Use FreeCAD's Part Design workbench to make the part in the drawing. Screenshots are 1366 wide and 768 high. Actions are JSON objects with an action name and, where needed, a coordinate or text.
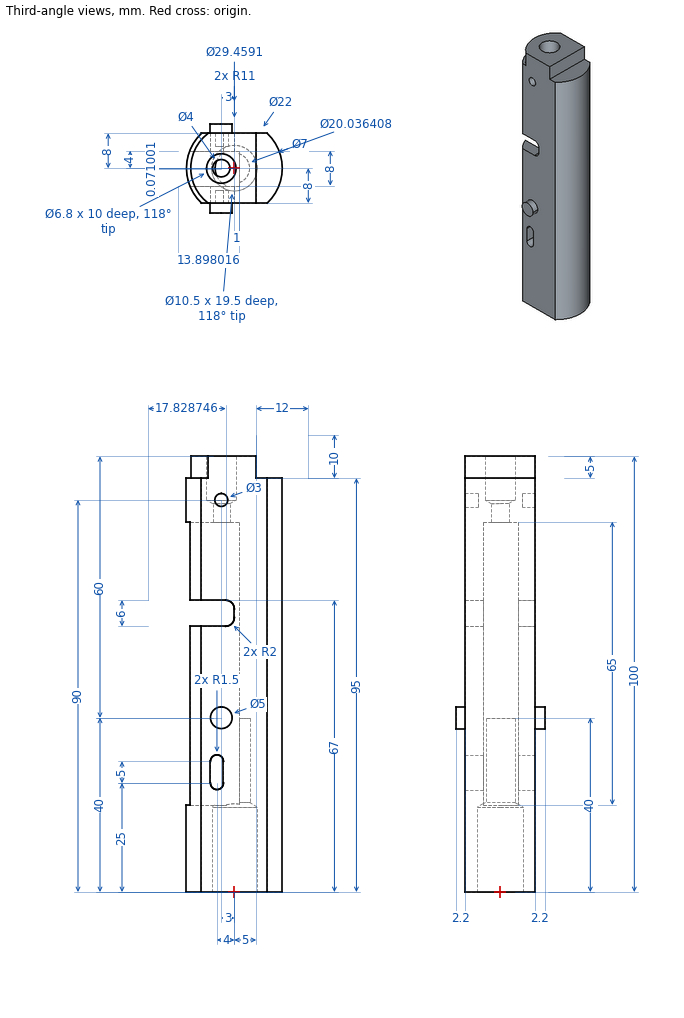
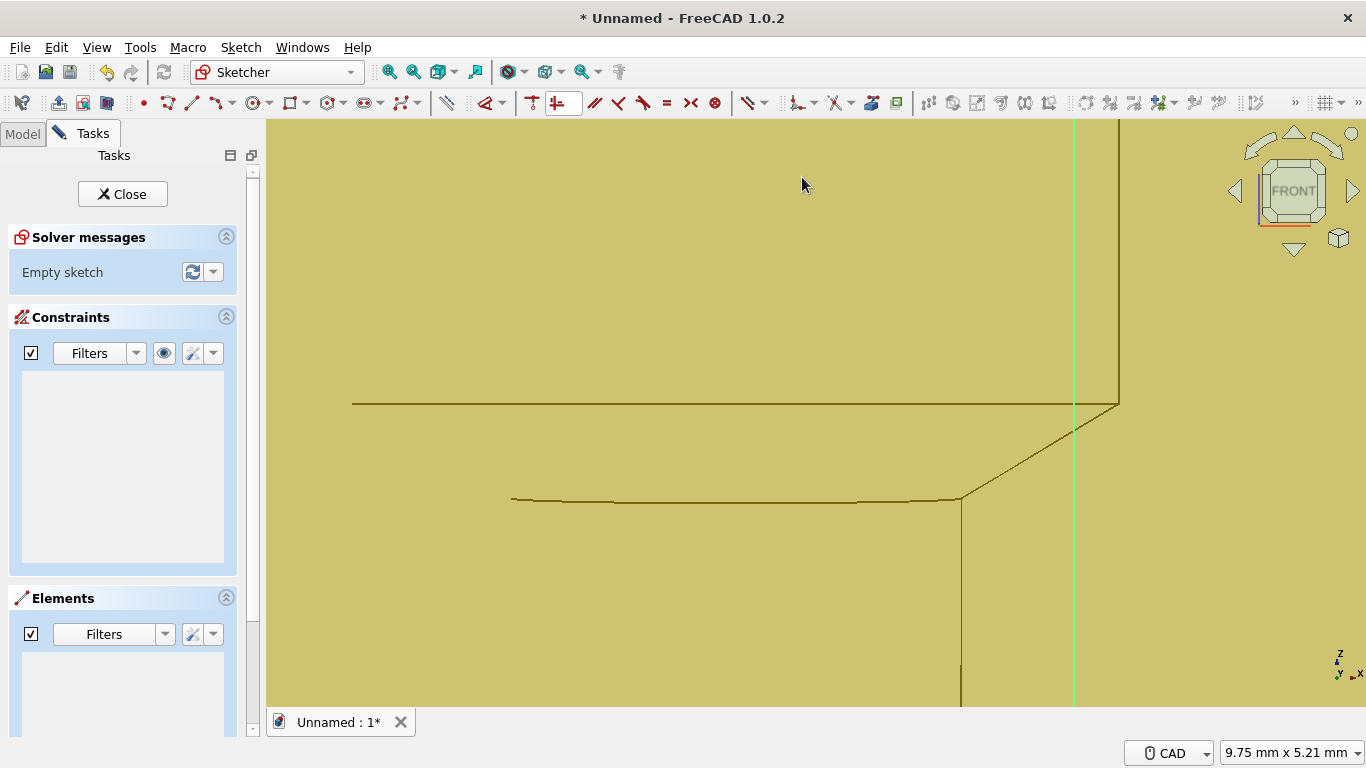
{"action": "key", "text": "g c"}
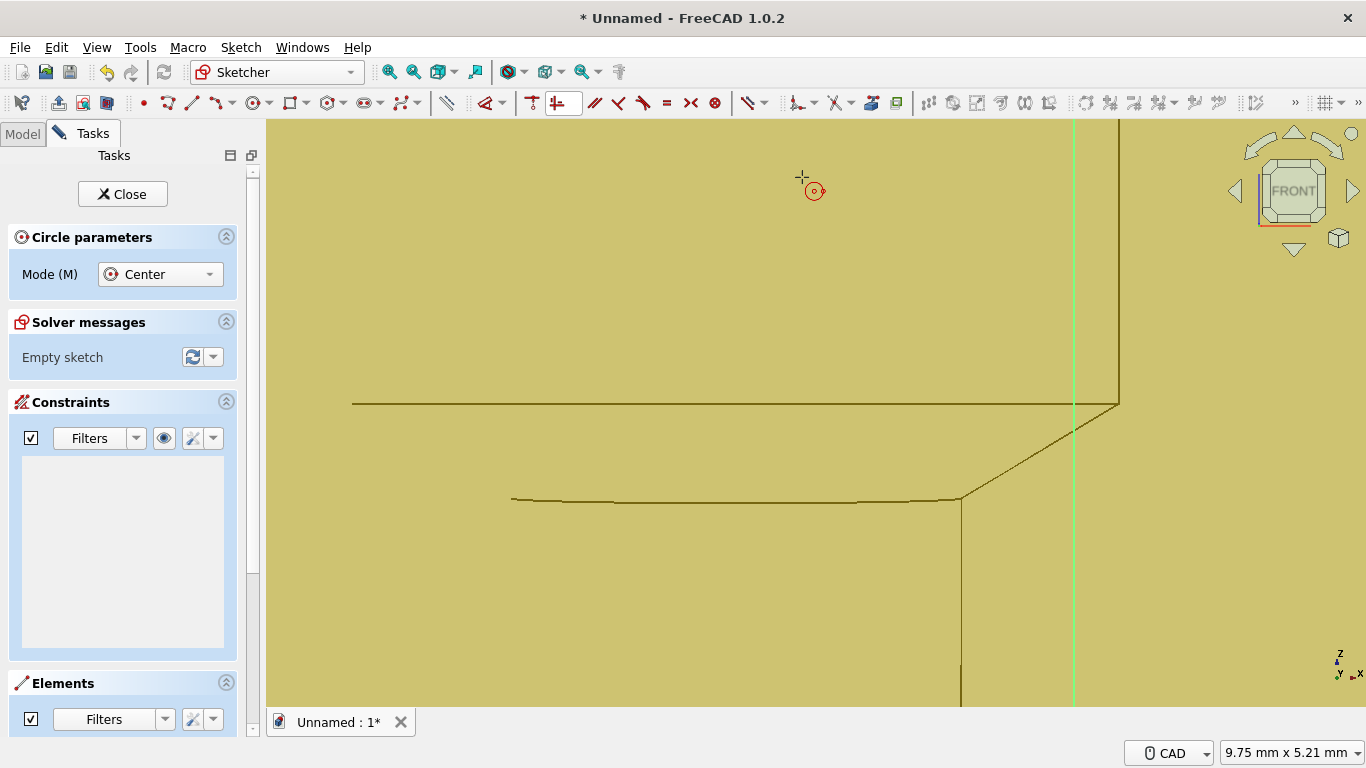
{"action": "left_click", "coordinate": [736, 404]}
{"action": "mouse_move", "coordinate": [855, 284]}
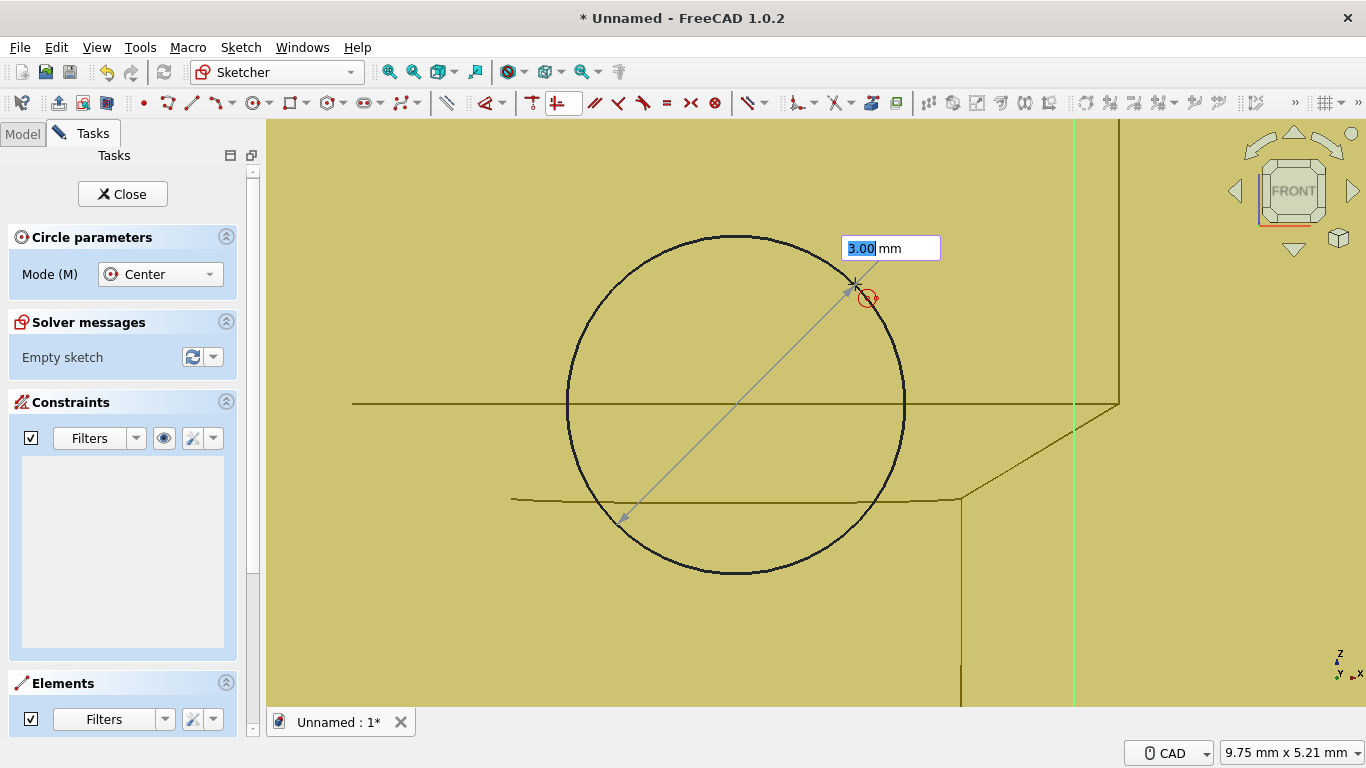
{"action": "type", "text": "3"}
{"action": "key", "text": "Return"}
{"action": "key", "text": "Escape"}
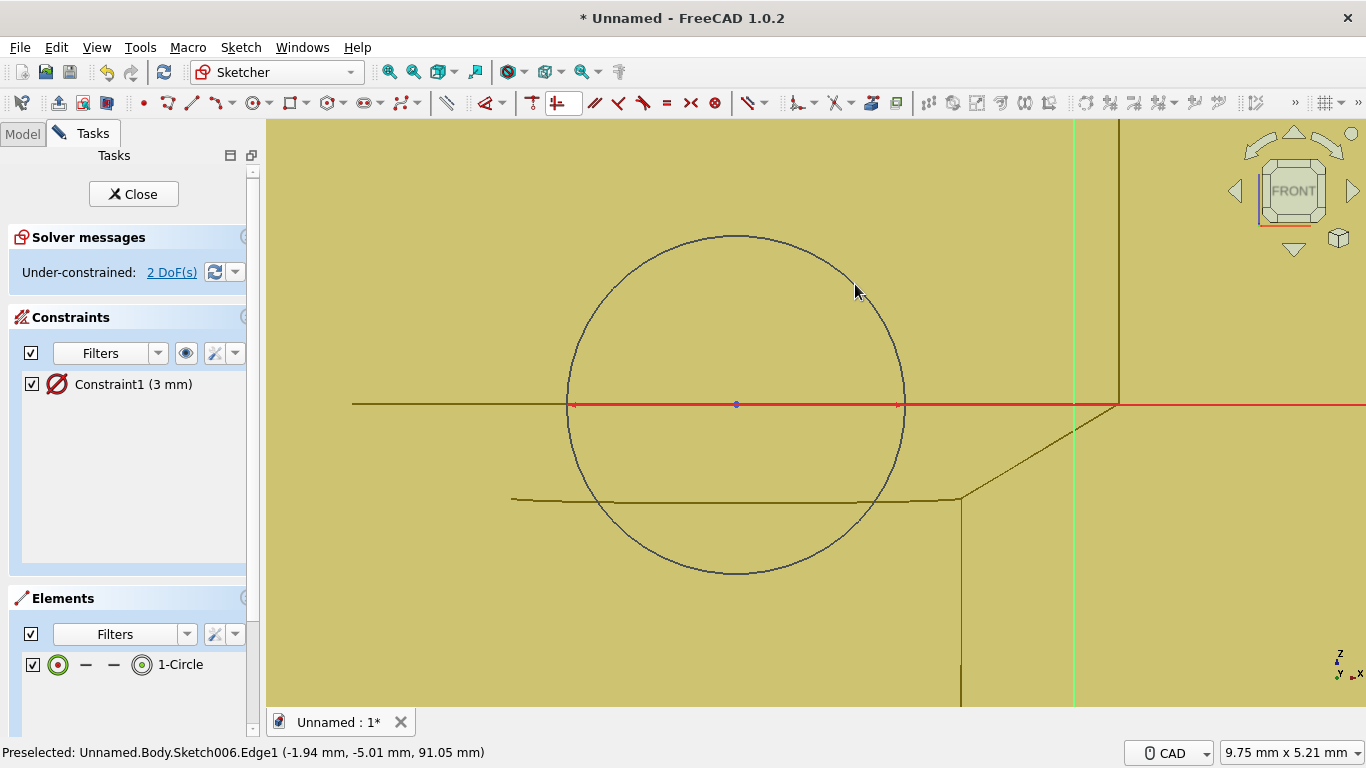
{"action": "left_click", "coordinate": [486, 104]}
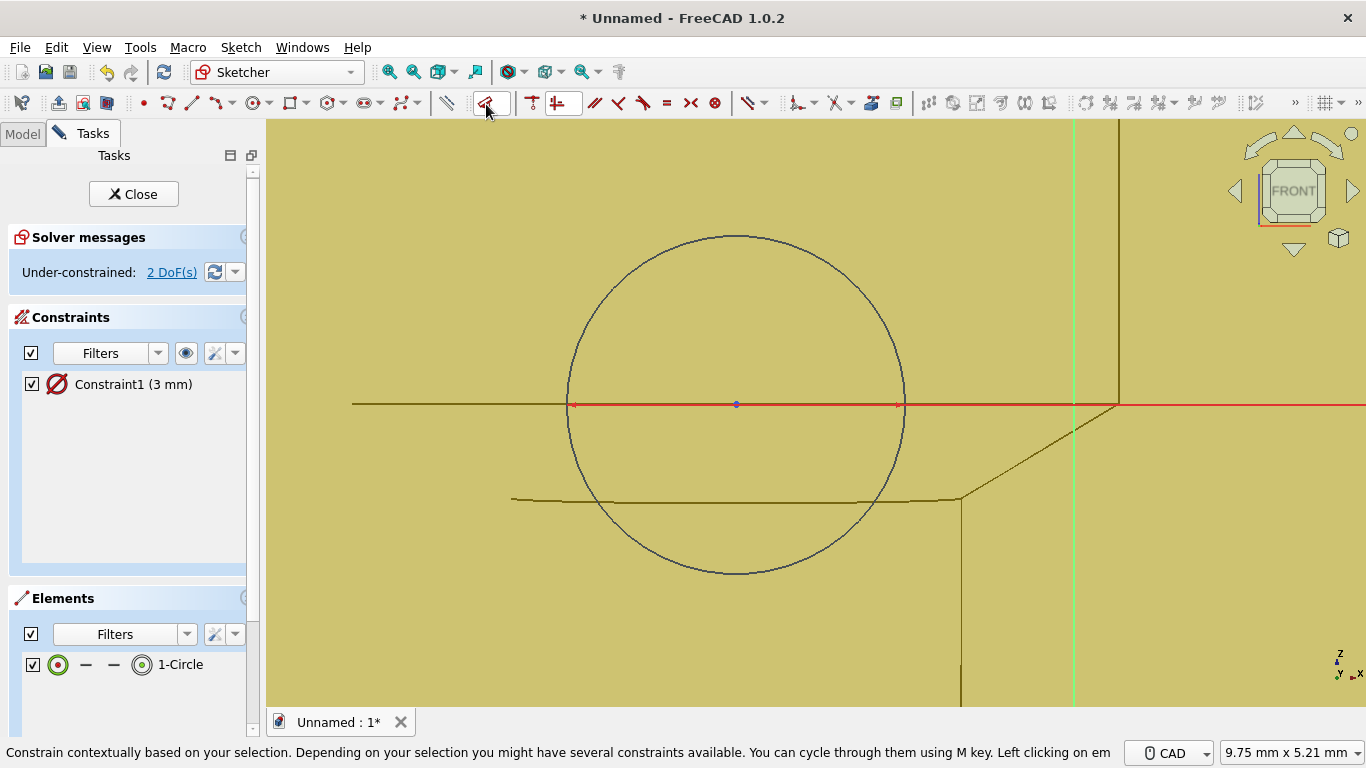
{"action": "left_click", "coordinate": [736, 405]}
{"action": "left_click", "coordinate": [827, 371]}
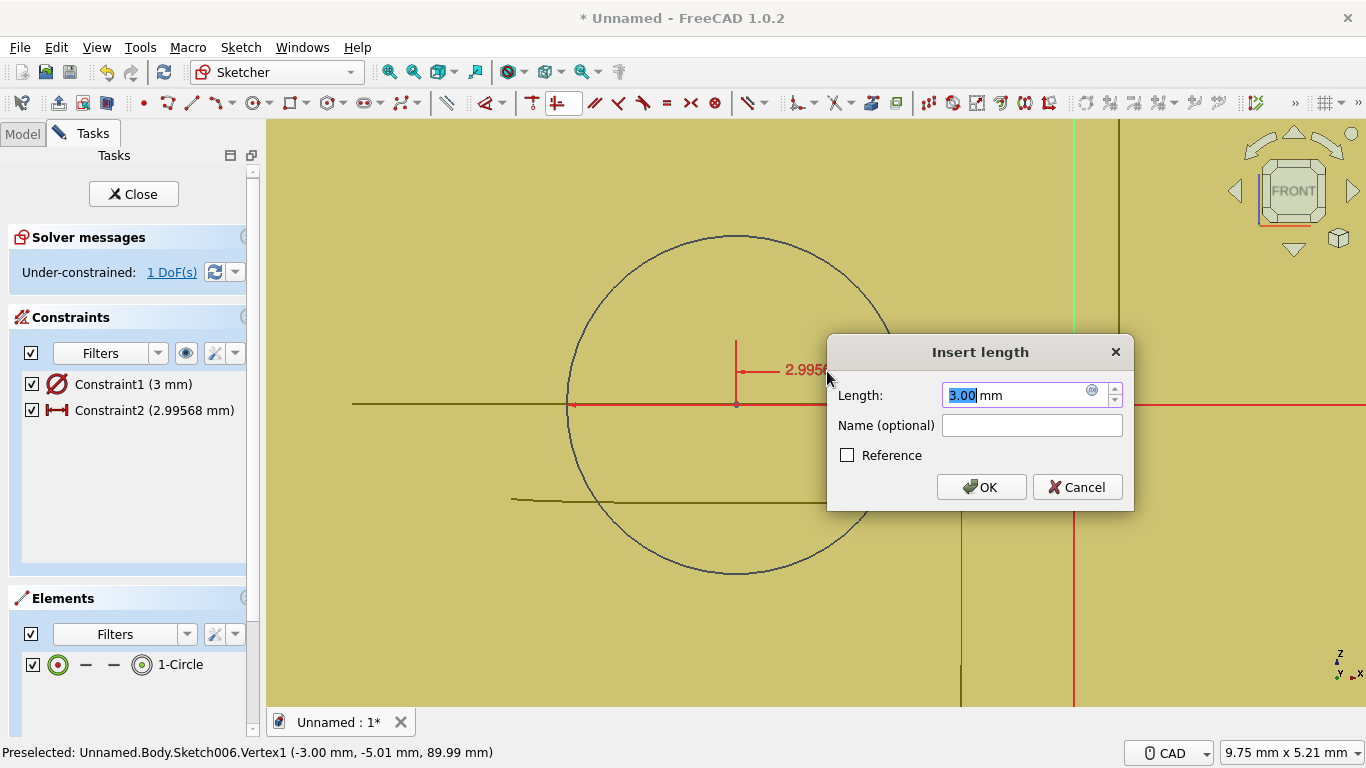
{"action": "type", "text": "3"}
{"action": "key", "text": "Return"}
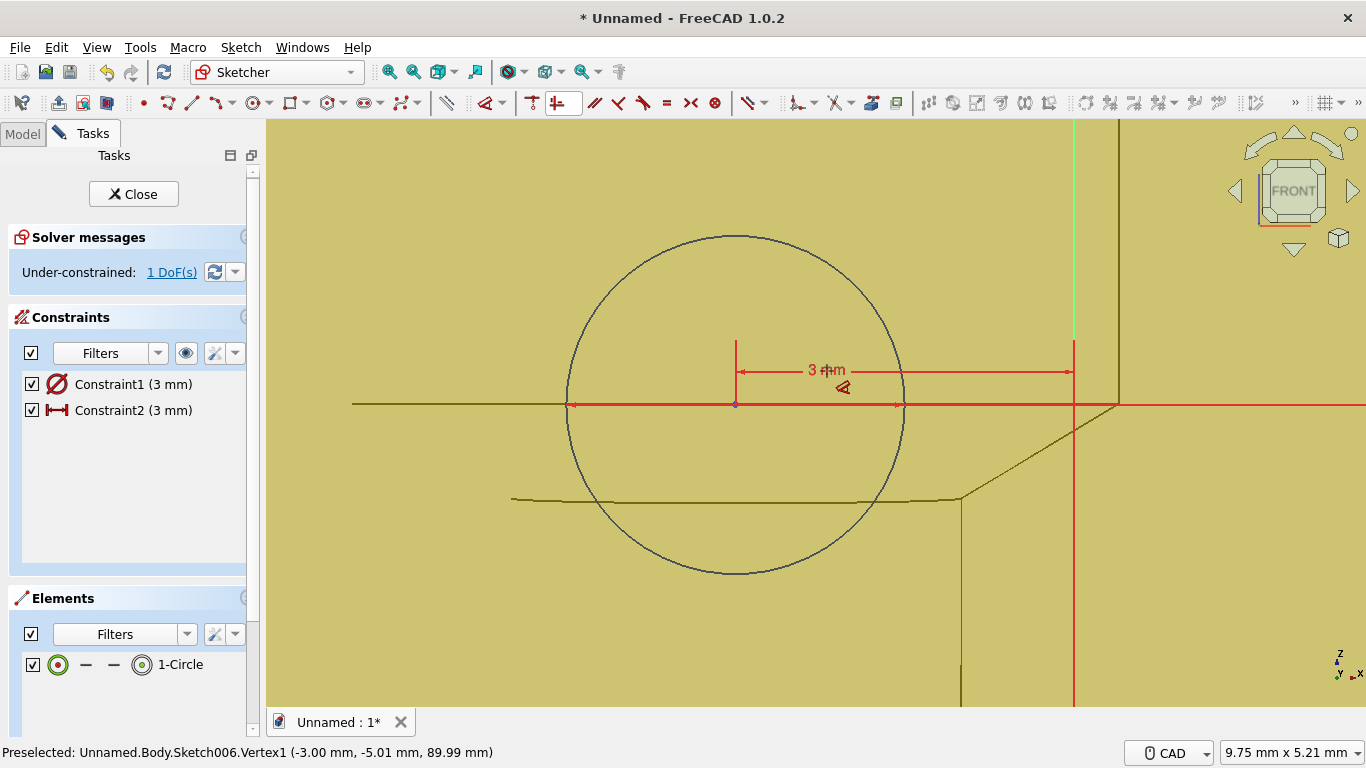
{"action": "left_click", "coordinate": [736, 405]}
{"action": "left_click", "coordinate": [1108, 542]}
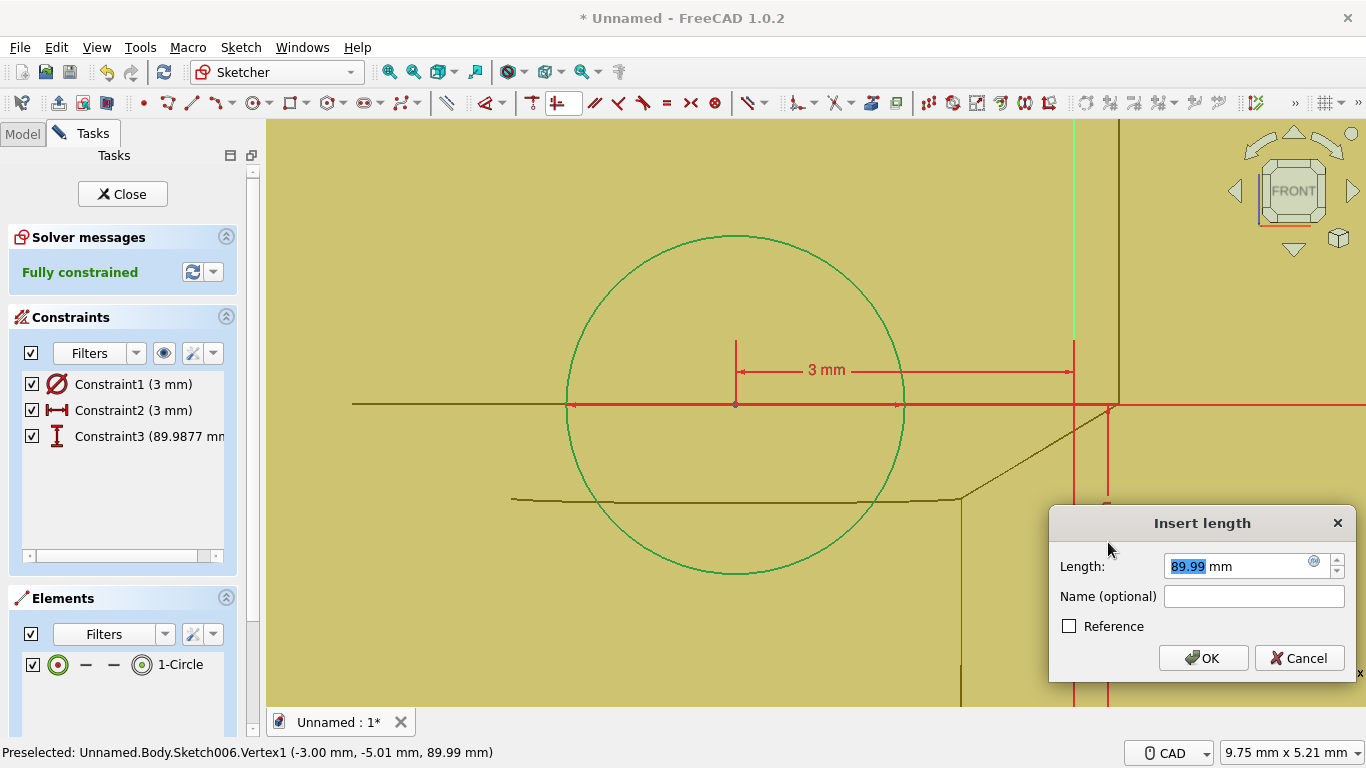
{"action": "type", "text": "90"}
{"action": "key", "text": "Return"}
{"action": "key", "text": "Escape"}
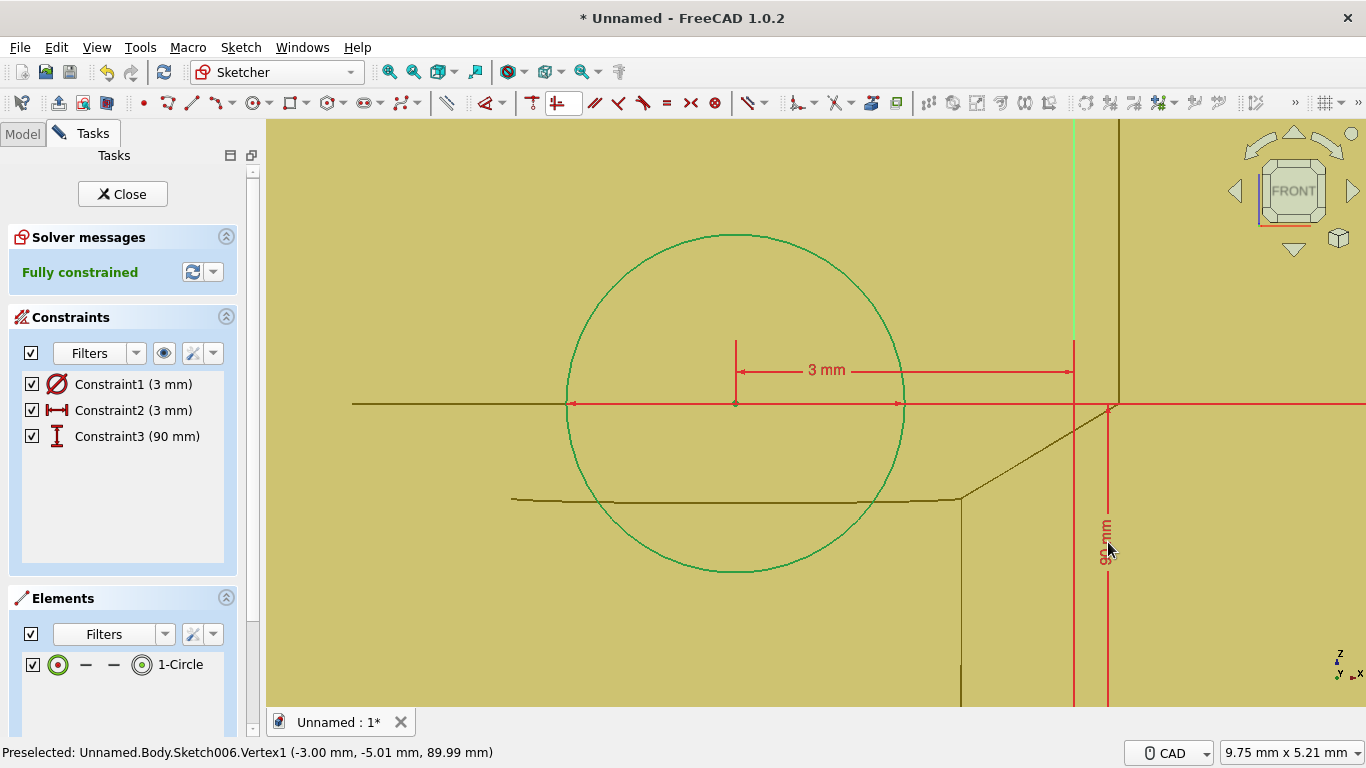
{"action": "left_click", "coordinate": [123, 194]}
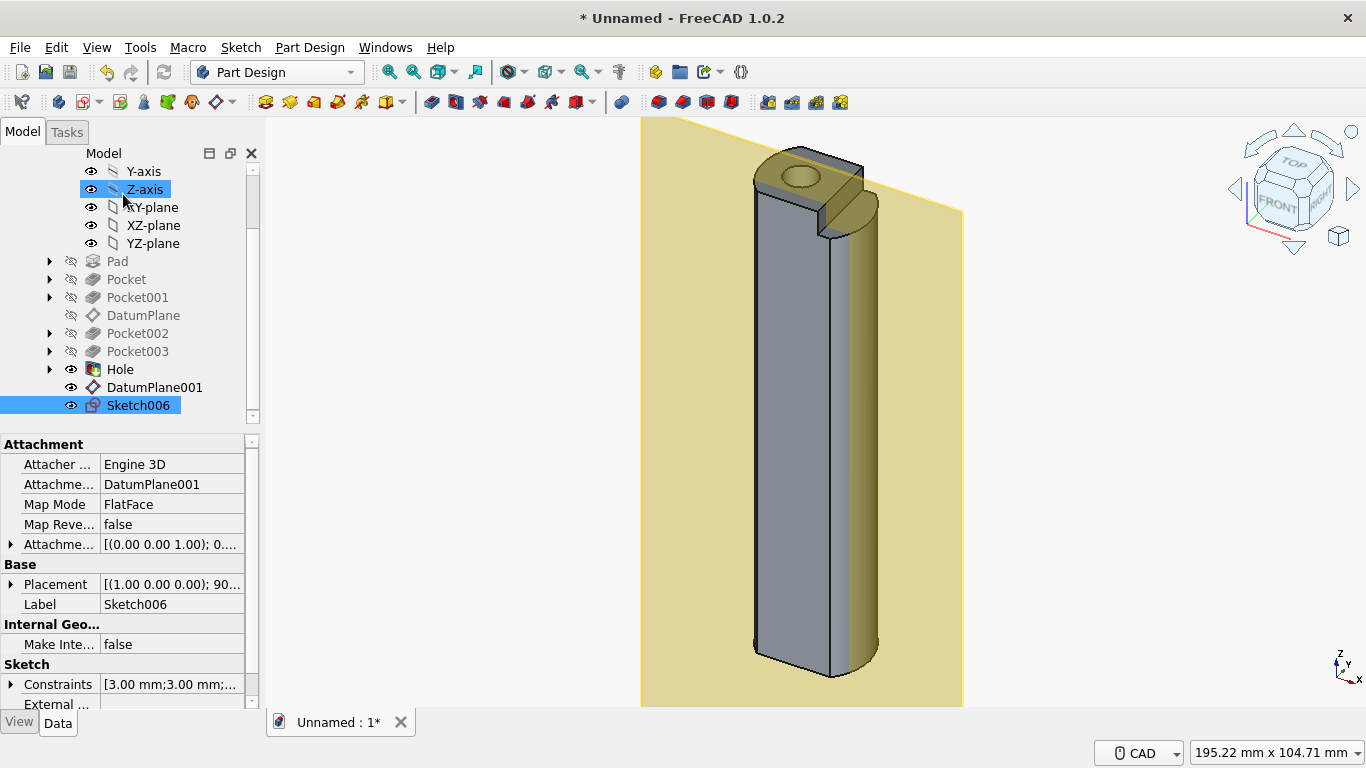
{"action": "left_click", "coordinate": [432, 102]}